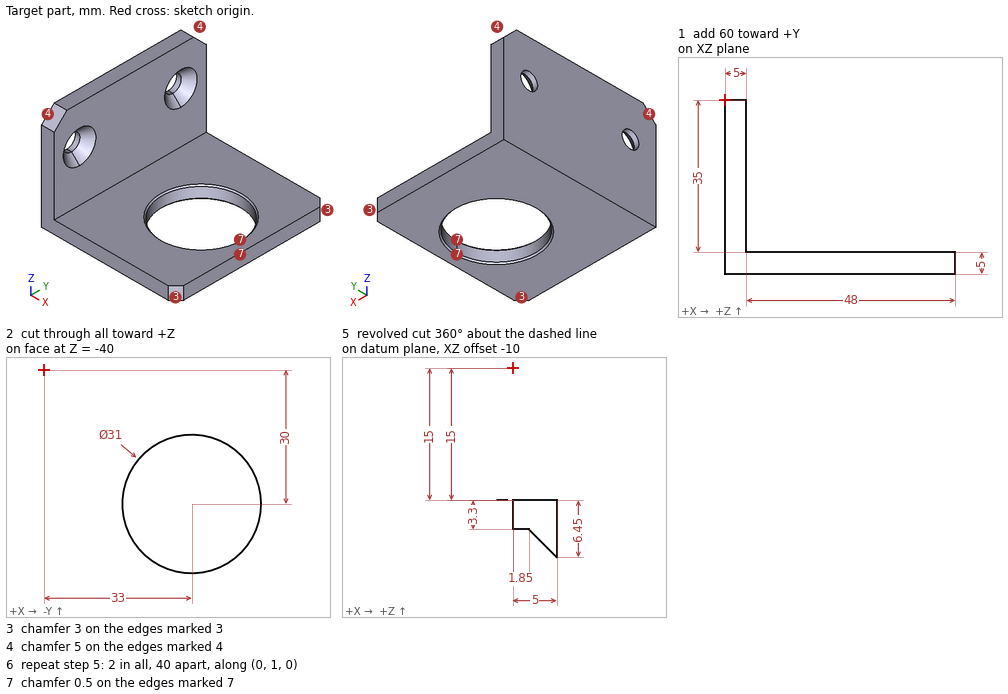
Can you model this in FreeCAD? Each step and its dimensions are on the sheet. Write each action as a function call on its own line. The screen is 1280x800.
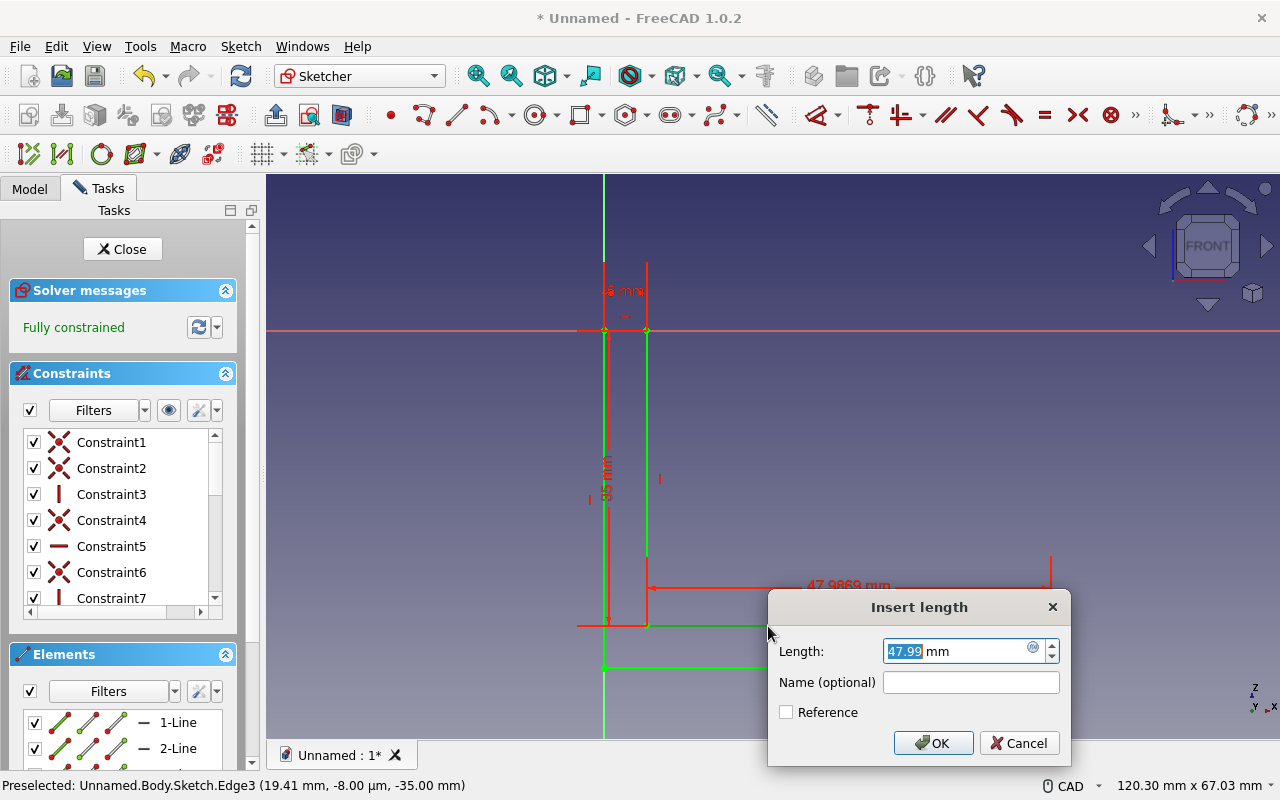
text(48)
key(Return)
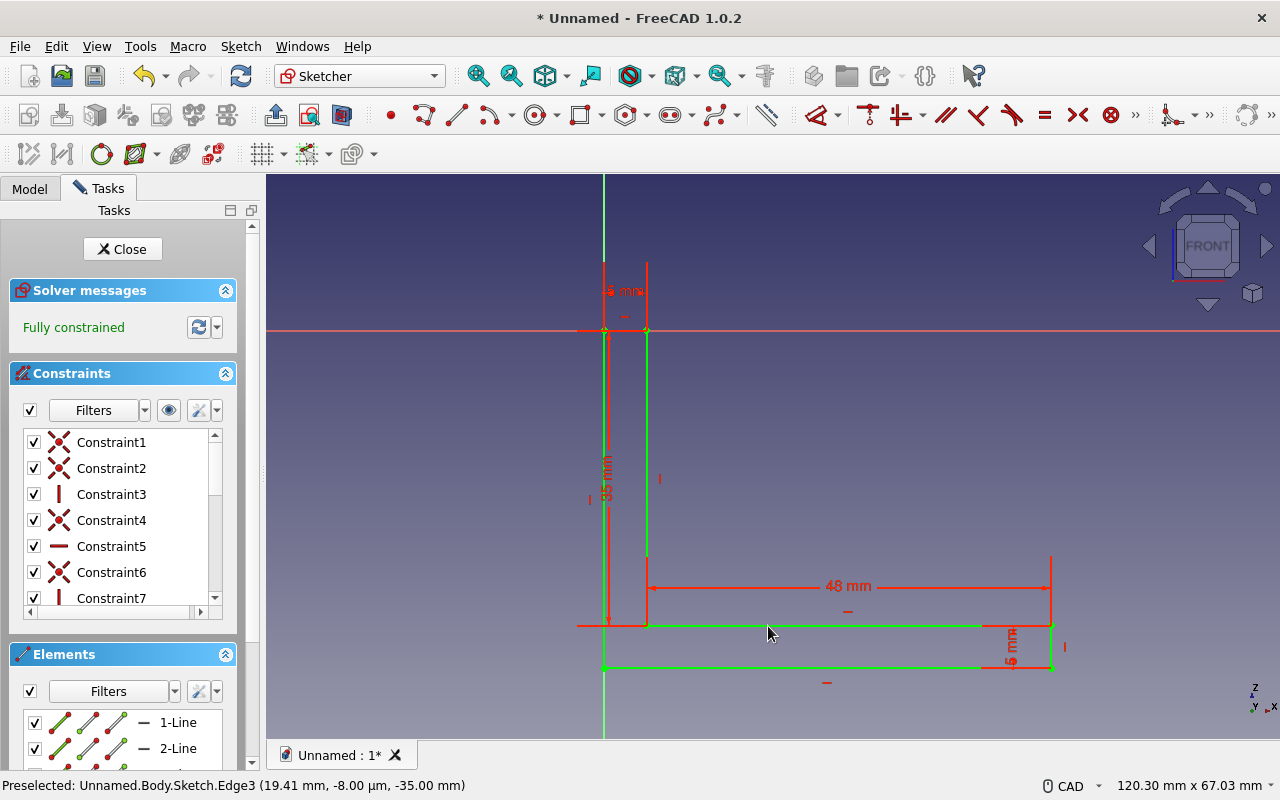
click(123, 249)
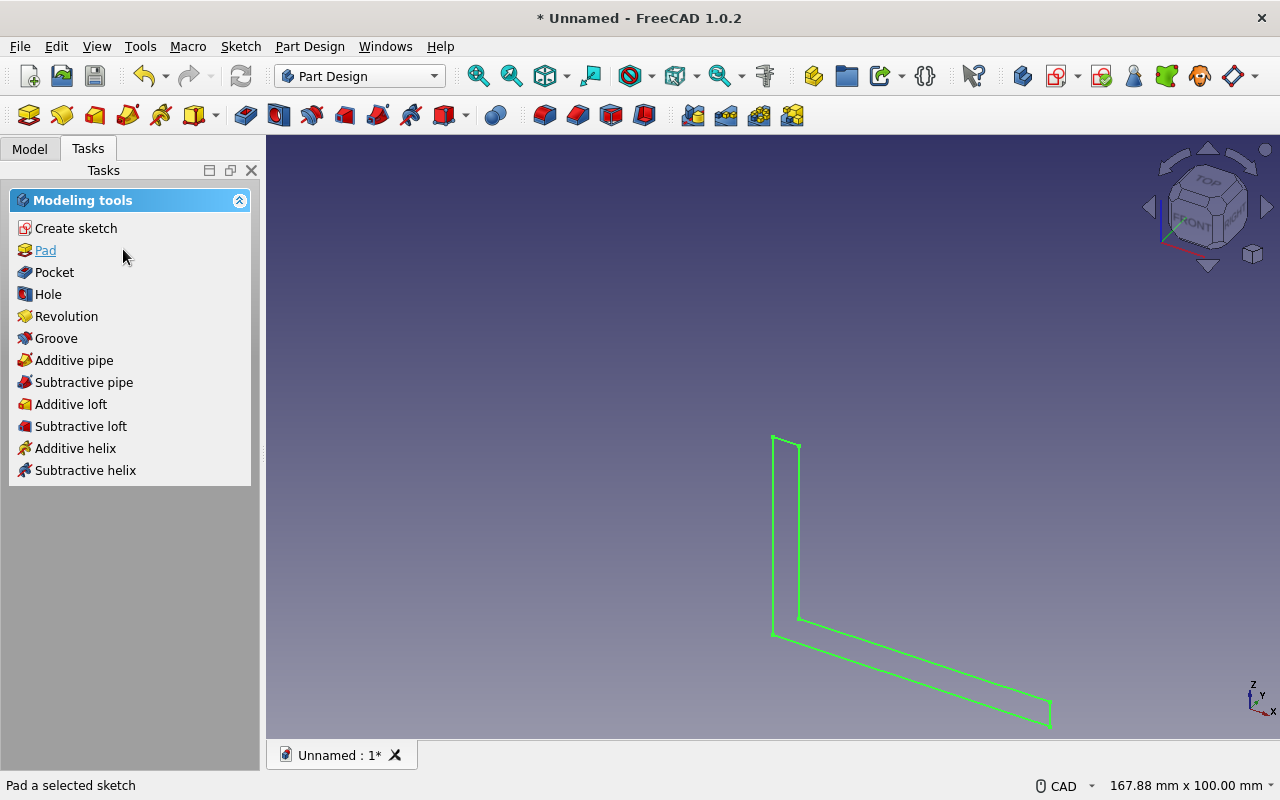
click(29, 116)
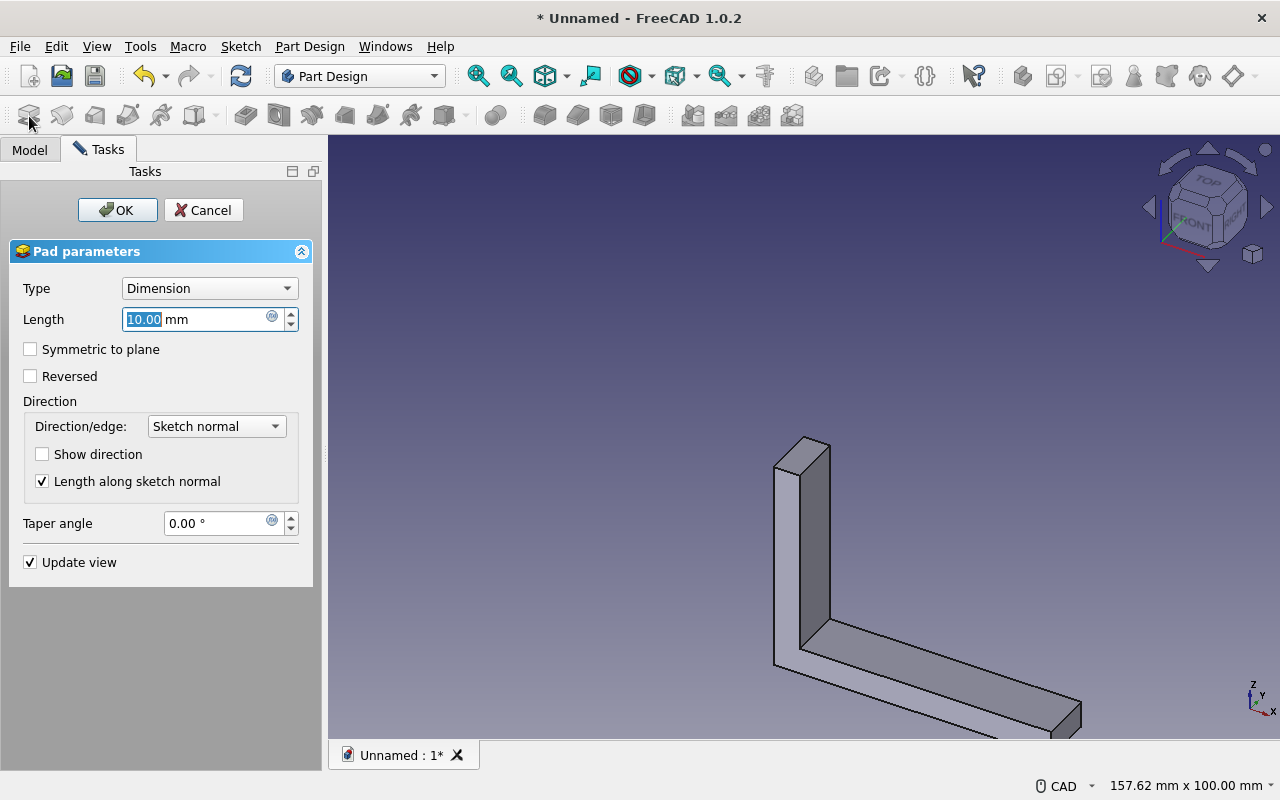
text(60)
key(Tab)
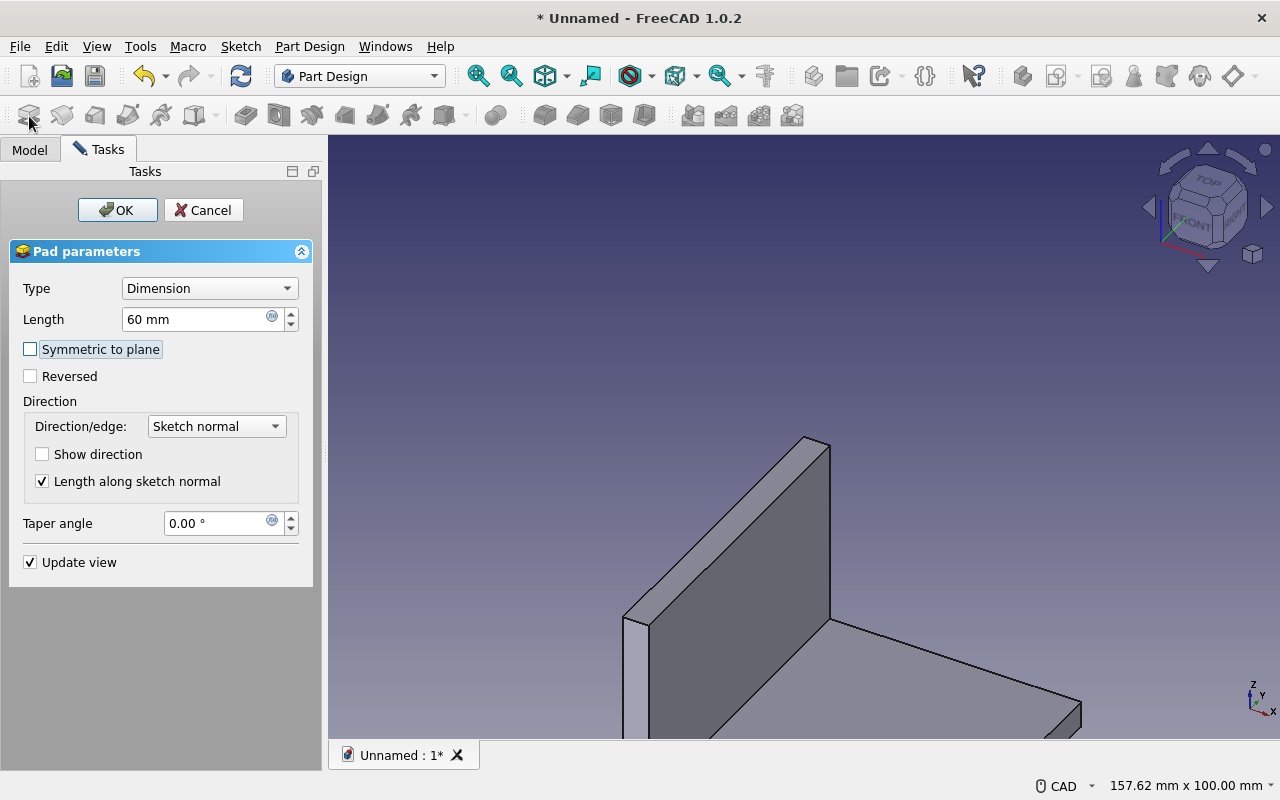
click(31, 376)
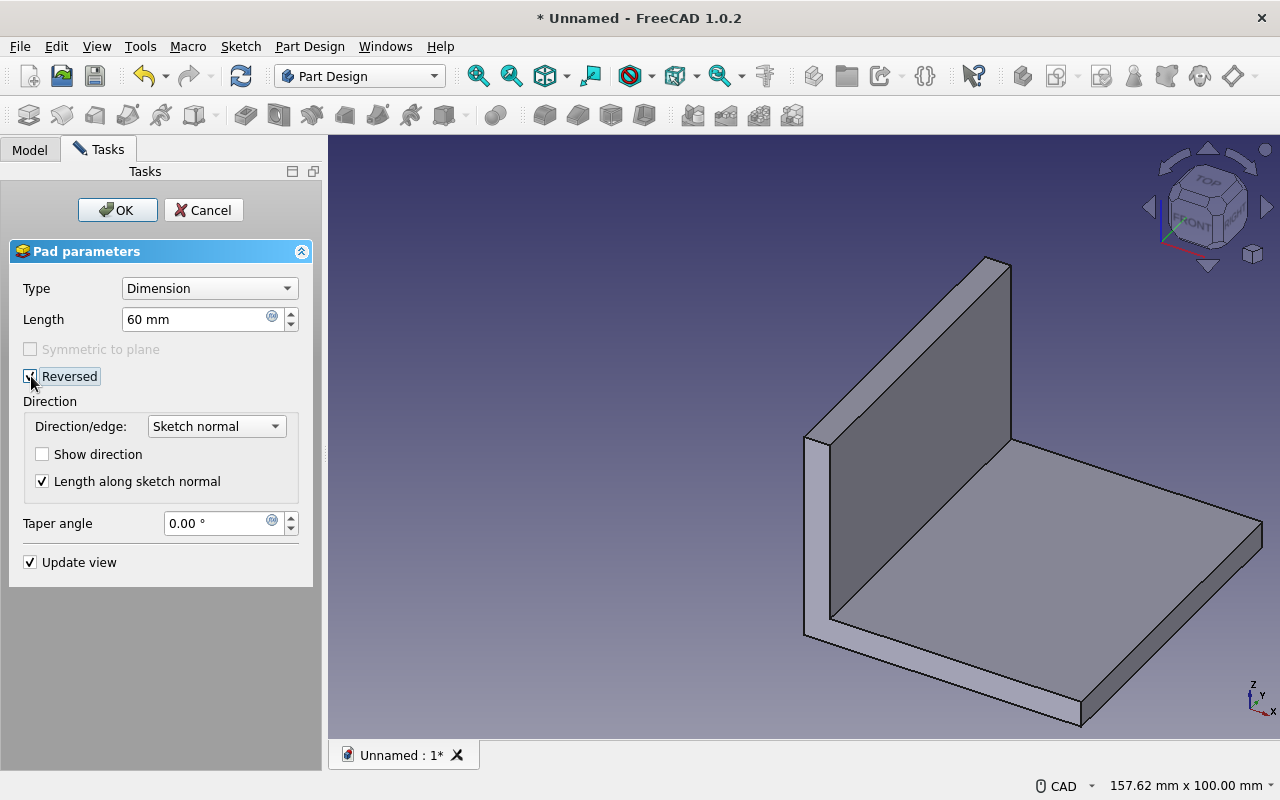
click(118, 210)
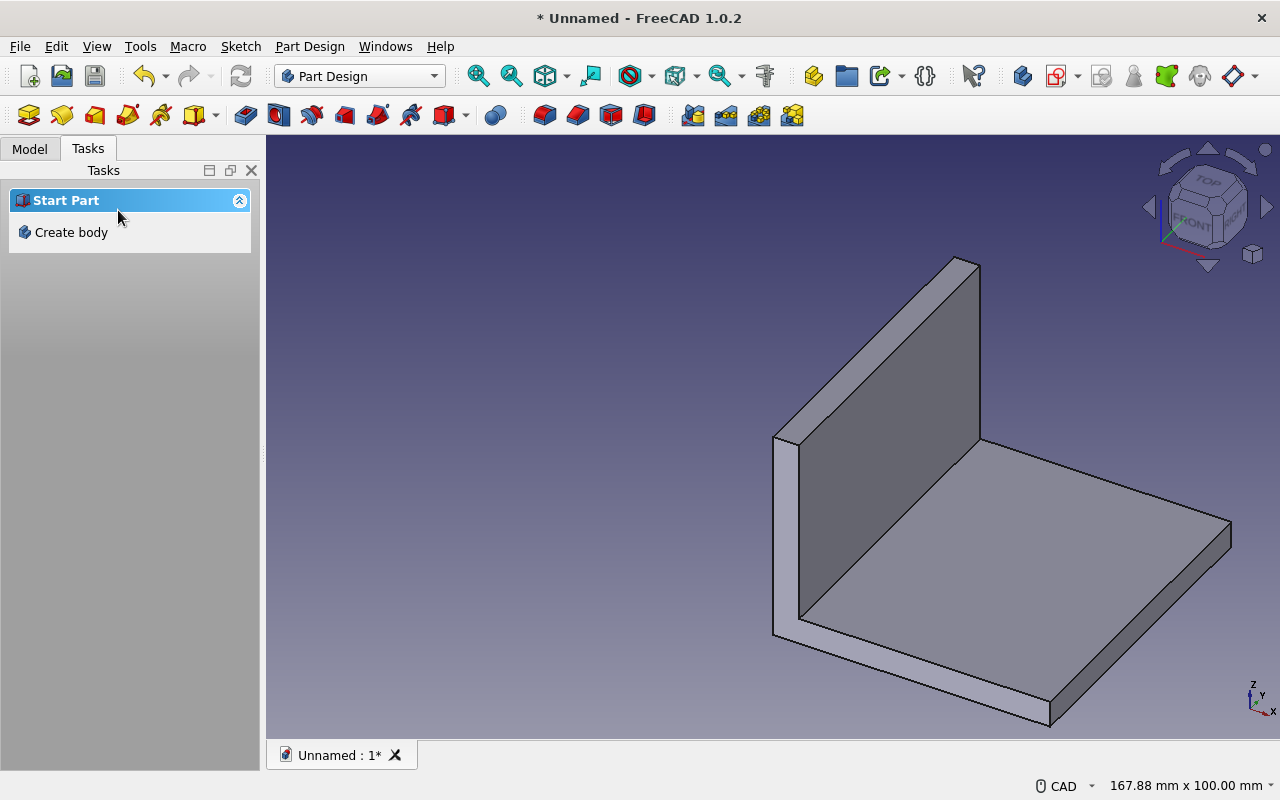
key(5)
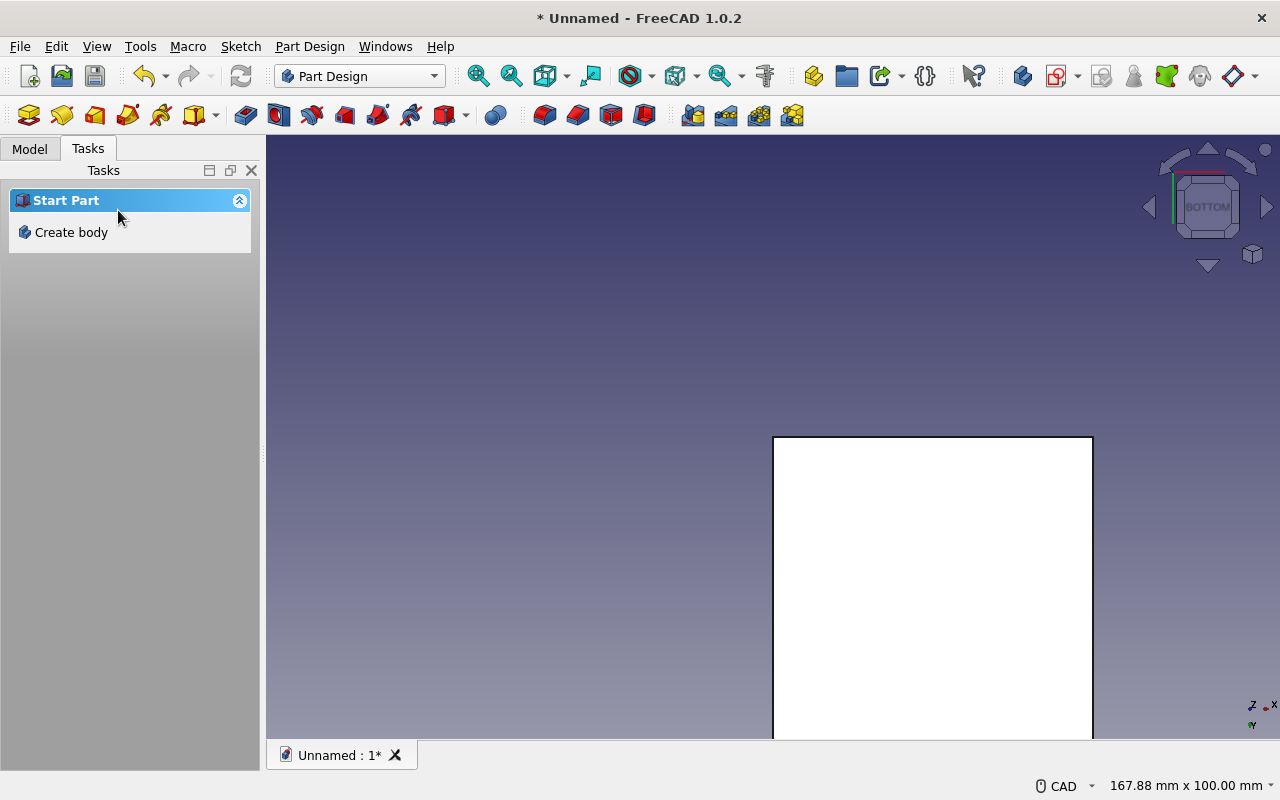
key(v)
key(f)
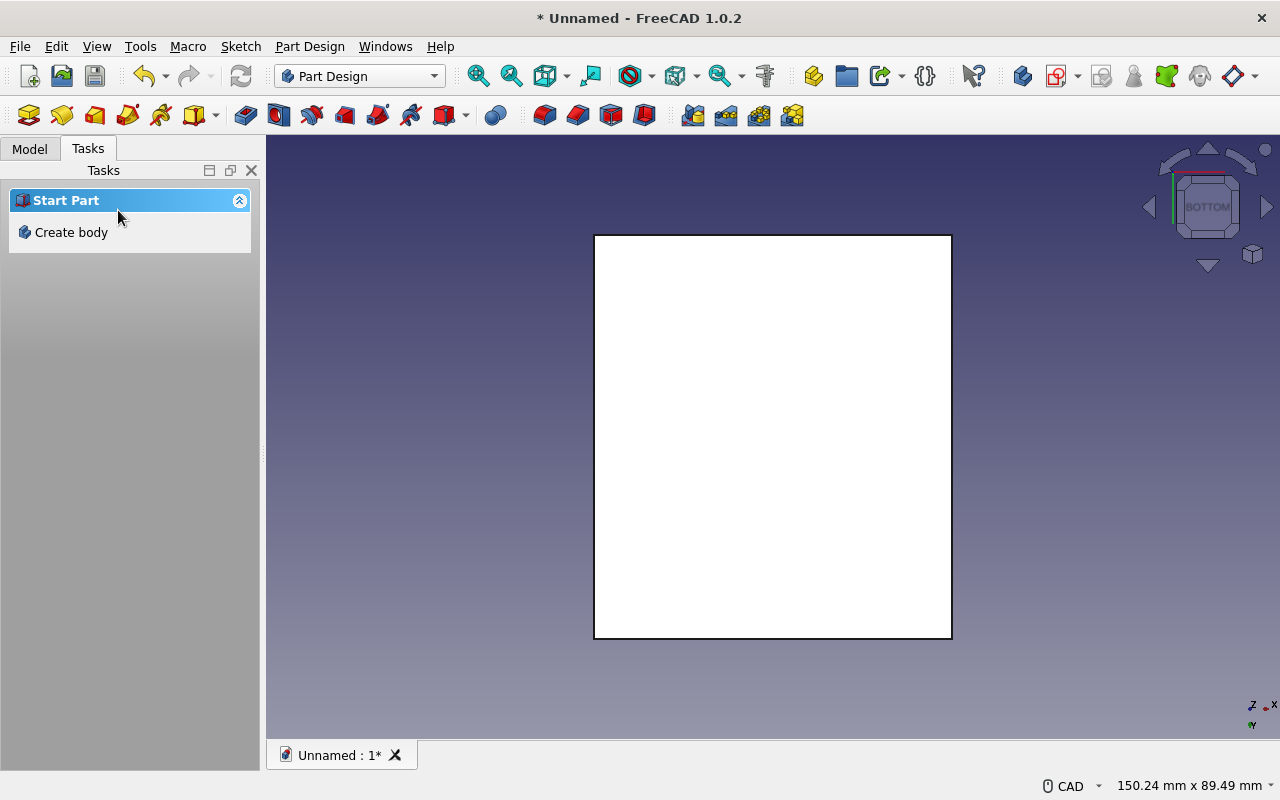
click(773, 436)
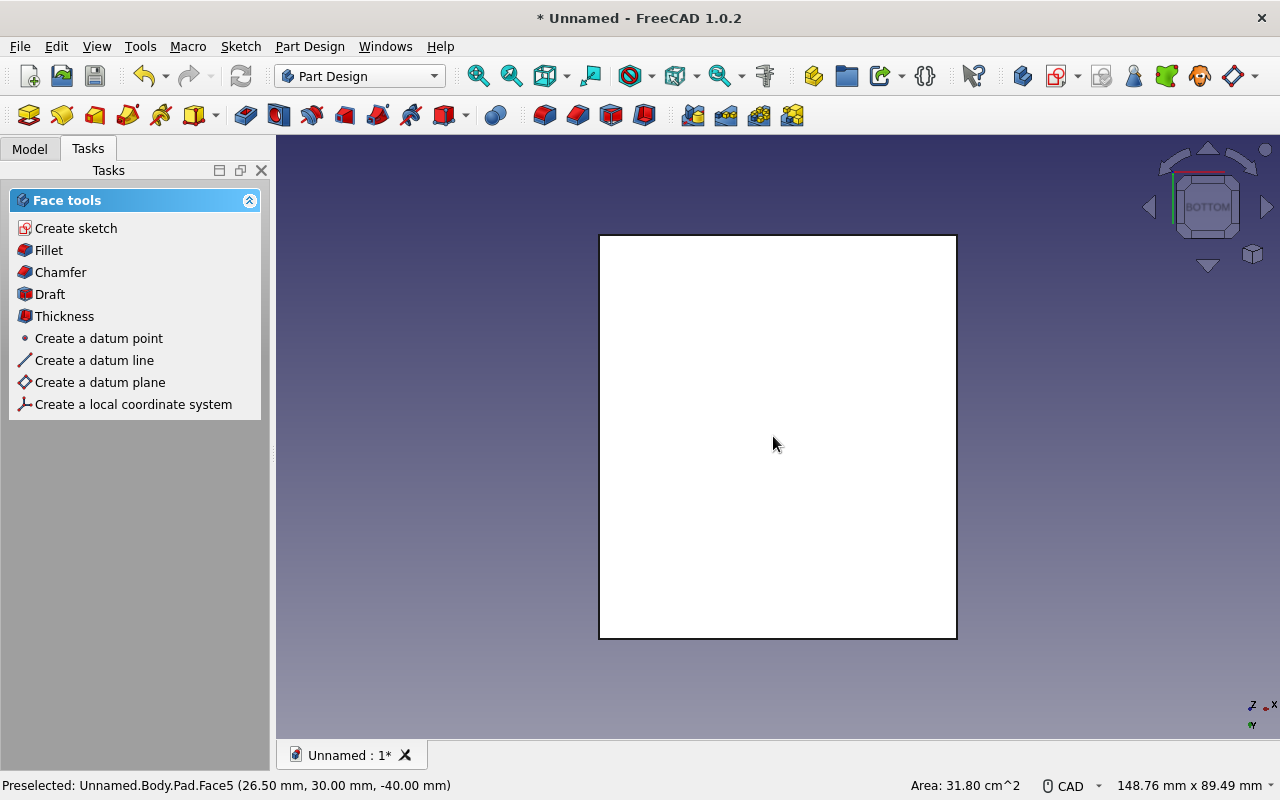
click(1056, 76)